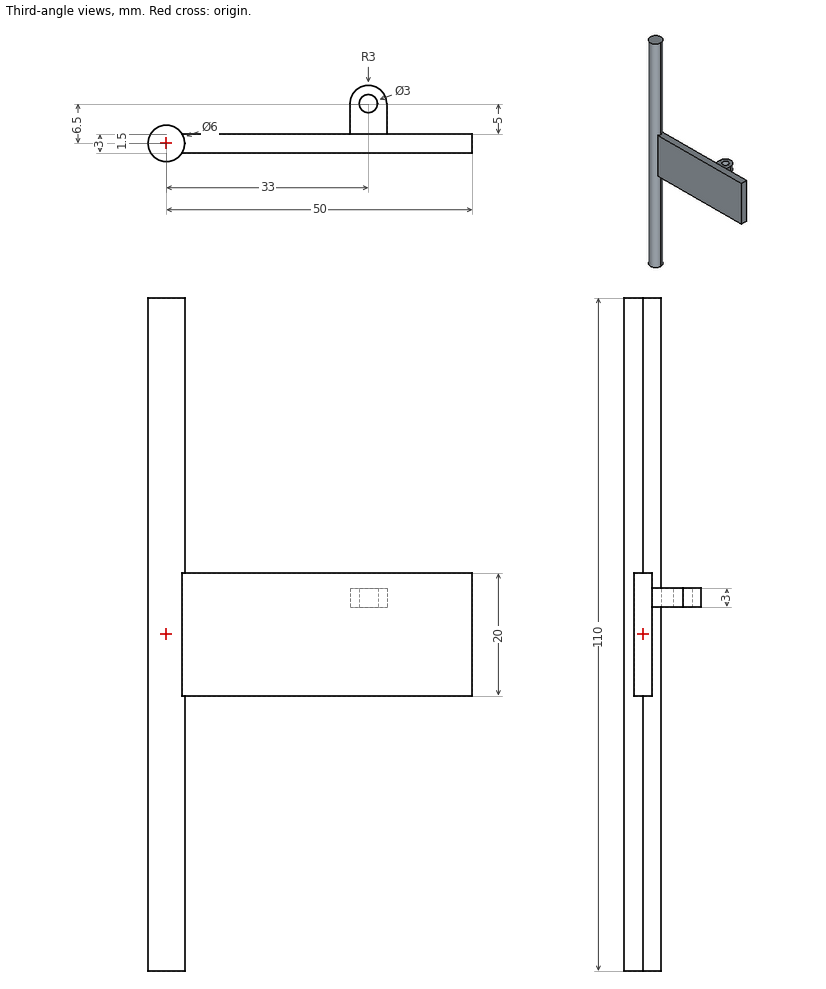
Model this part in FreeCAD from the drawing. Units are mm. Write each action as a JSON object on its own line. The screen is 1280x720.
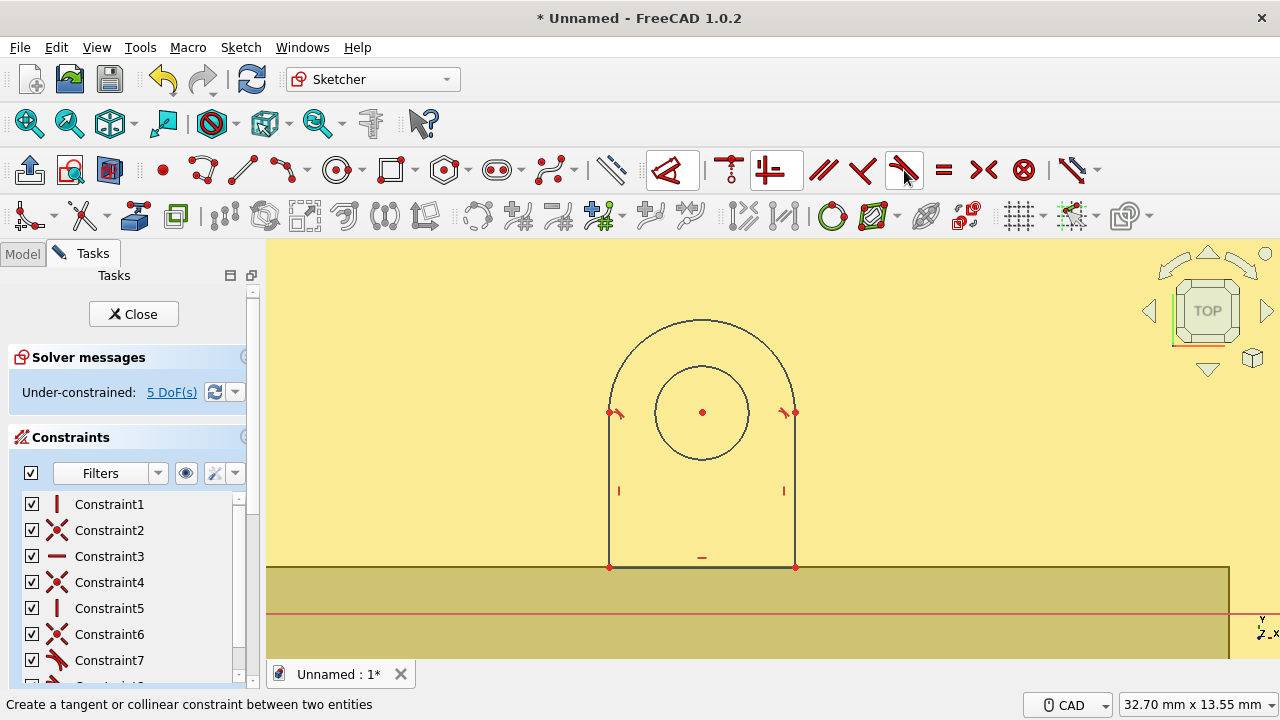
{"action": "left_click", "coordinate": [757, 338]}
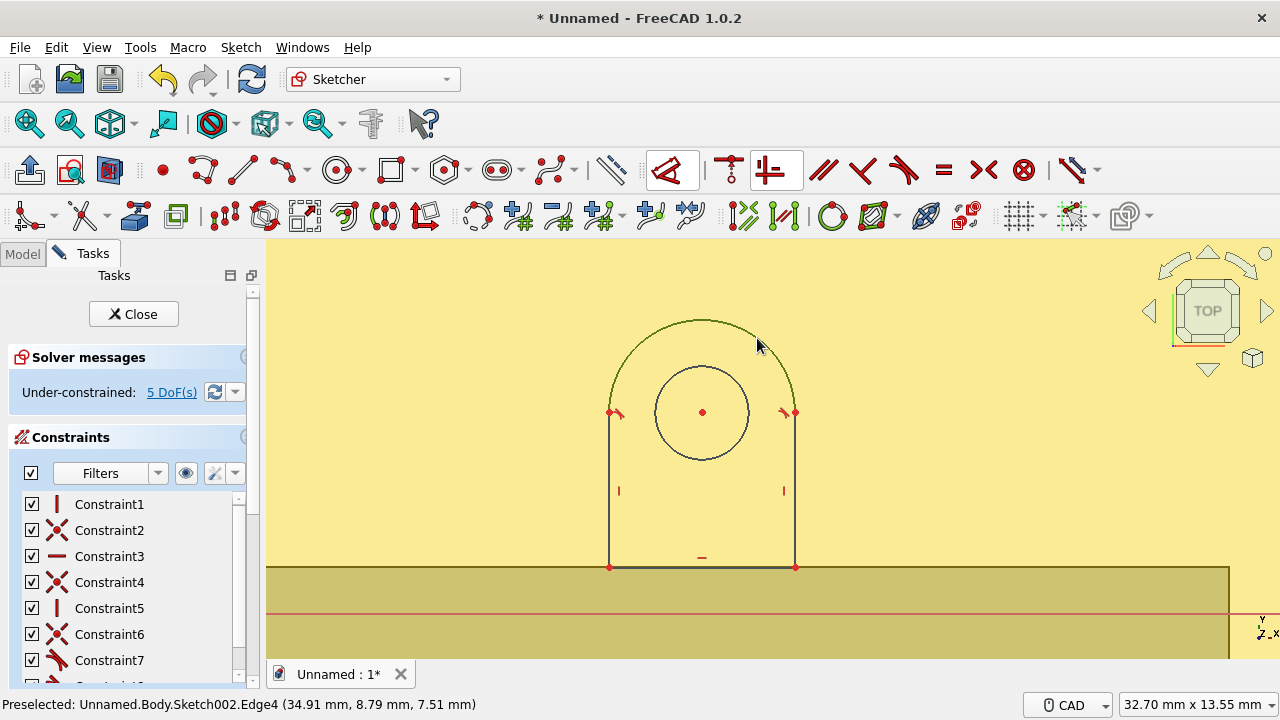
{"action": "left_click", "coordinate": [694, 170]}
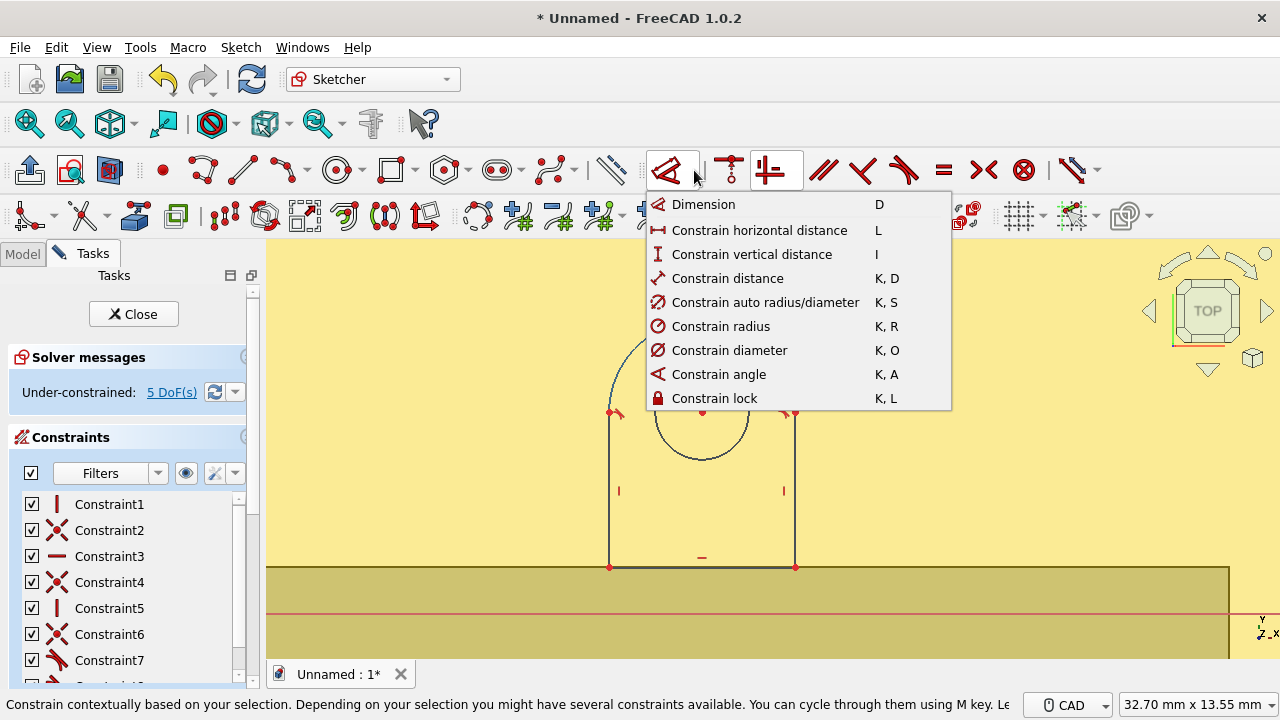
{"action": "left_click", "coordinate": [799, 326]}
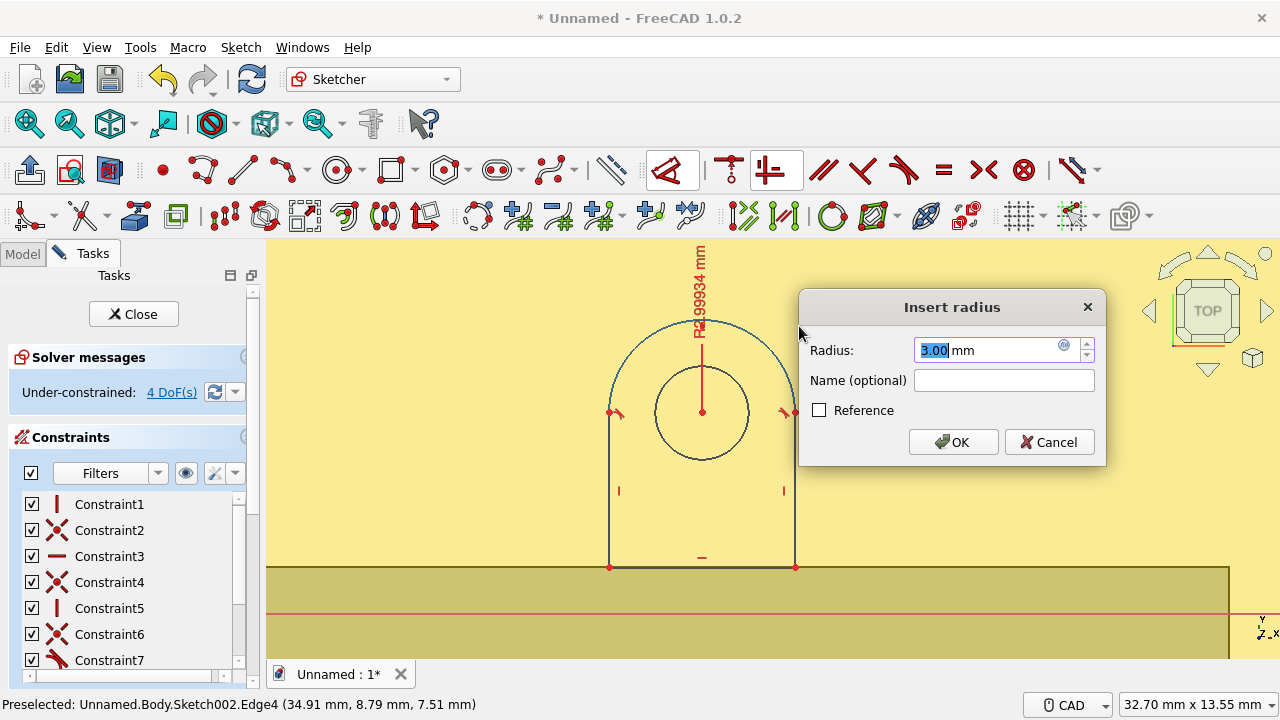
{"action": "type", "text": "3"}
{"action": "key", "text": "Return"}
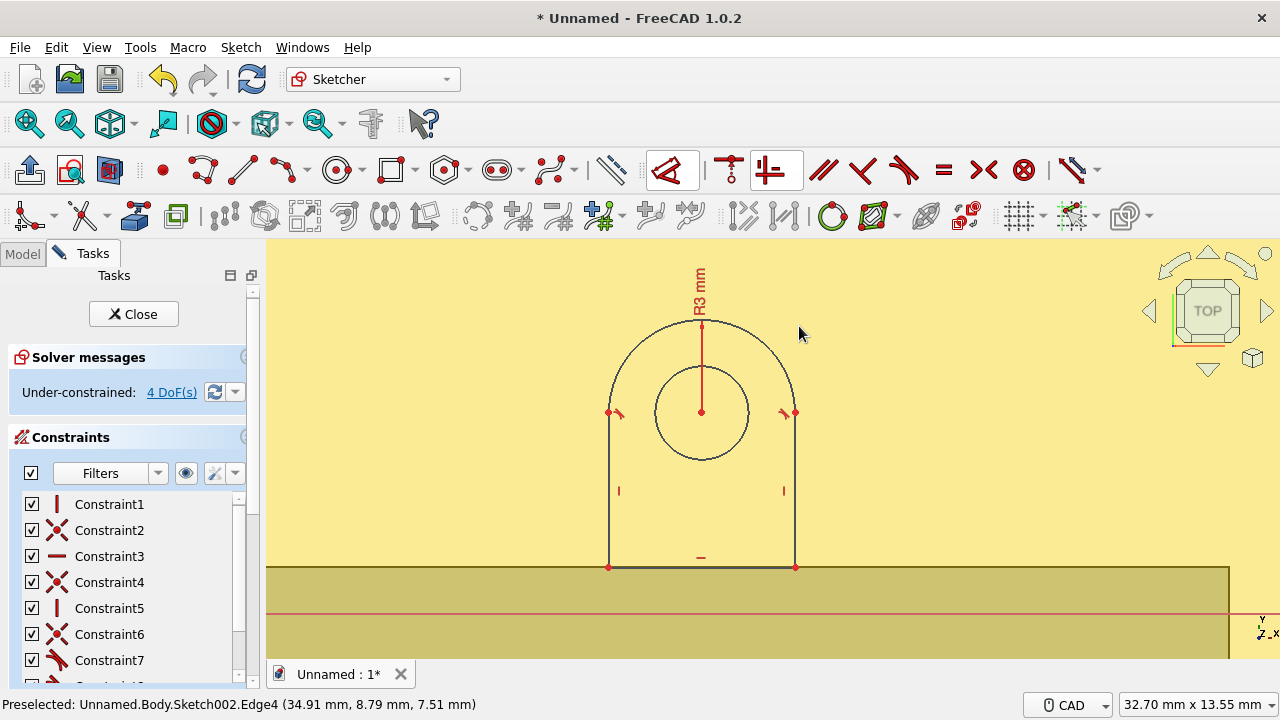
{"action": "left_click", "coordinate": [735, 380]}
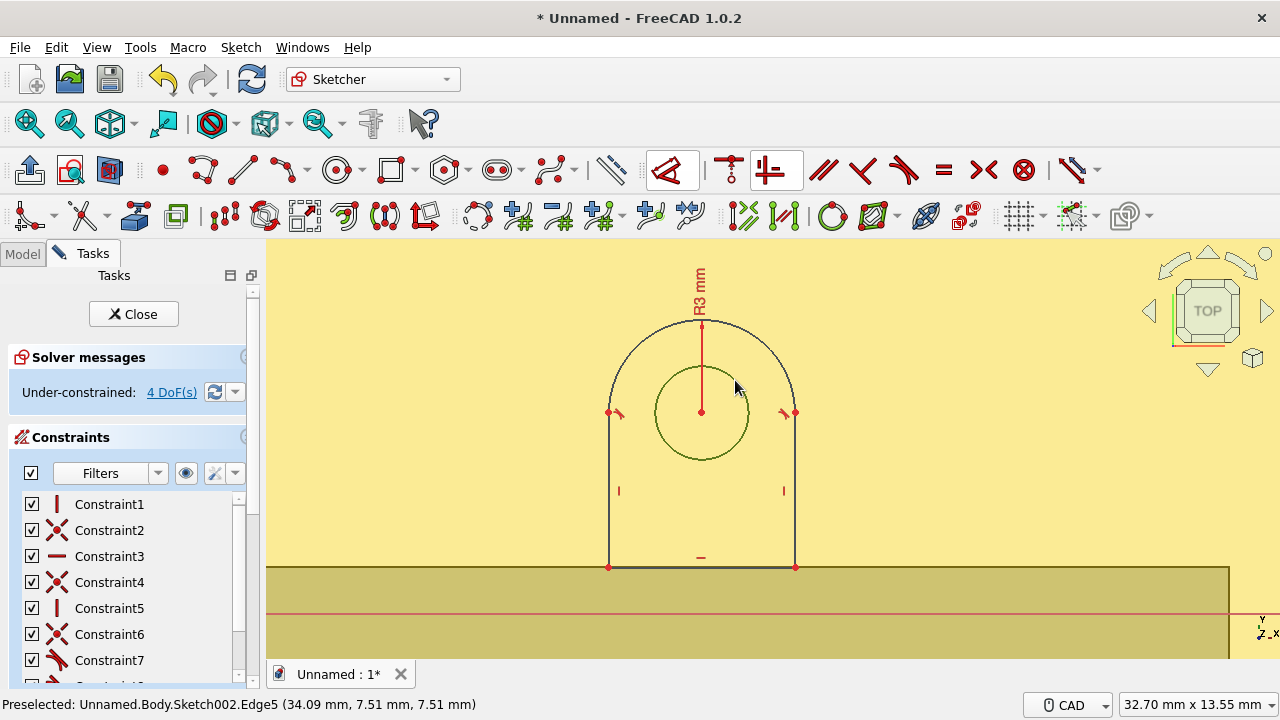
{"action": "left_click", "coordinate": [694, 170]}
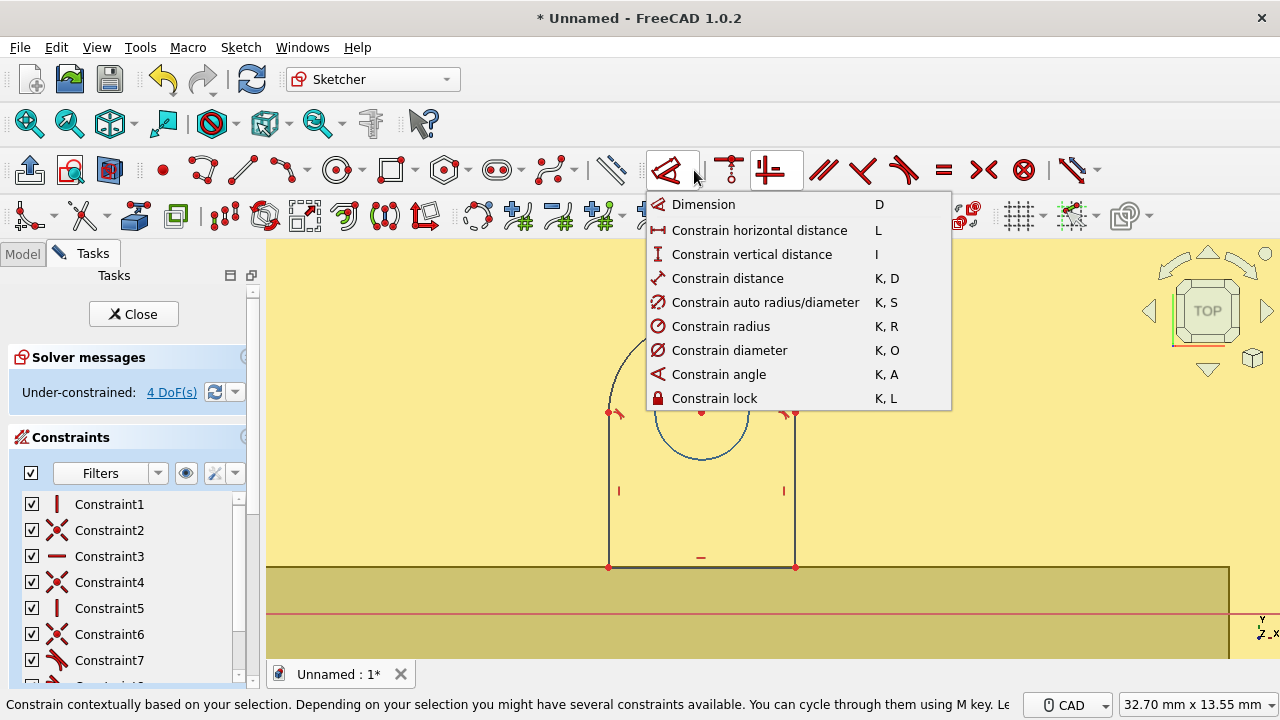
{"action": "left_click", "coordinate": [799, 350]}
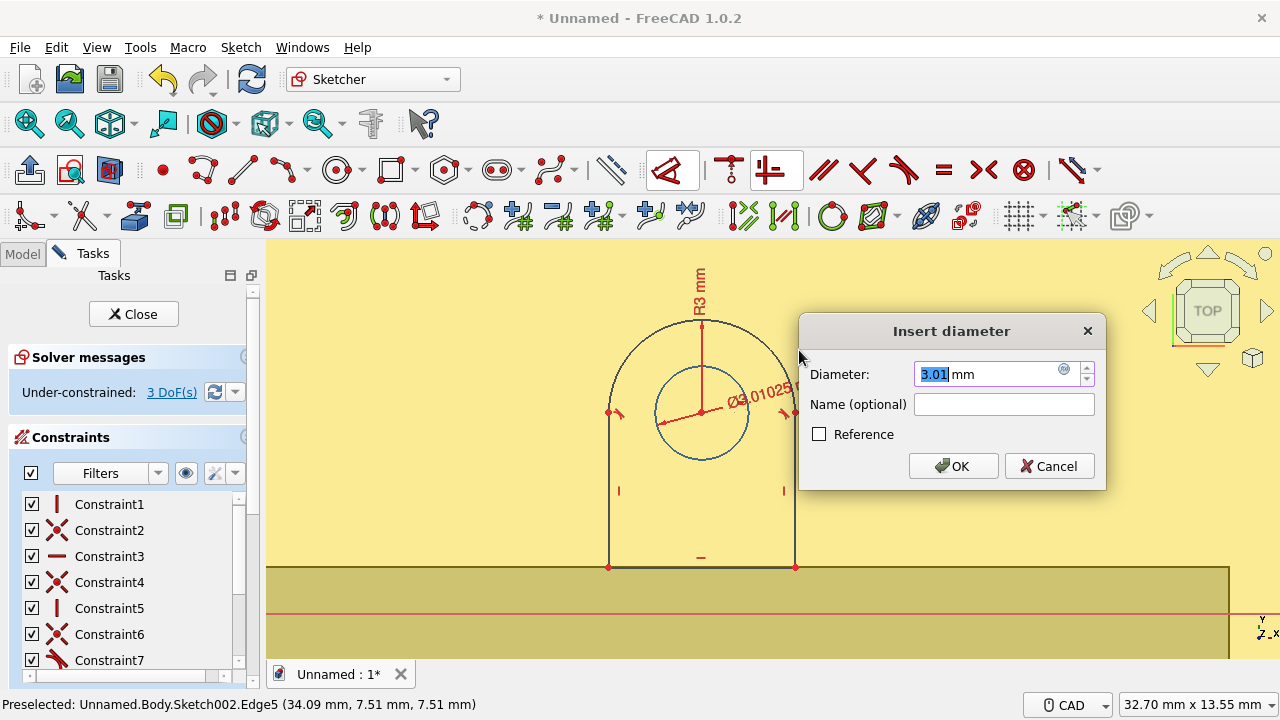
{"action": "type", "text": "3"}
{"action": "key", "text": "Return"}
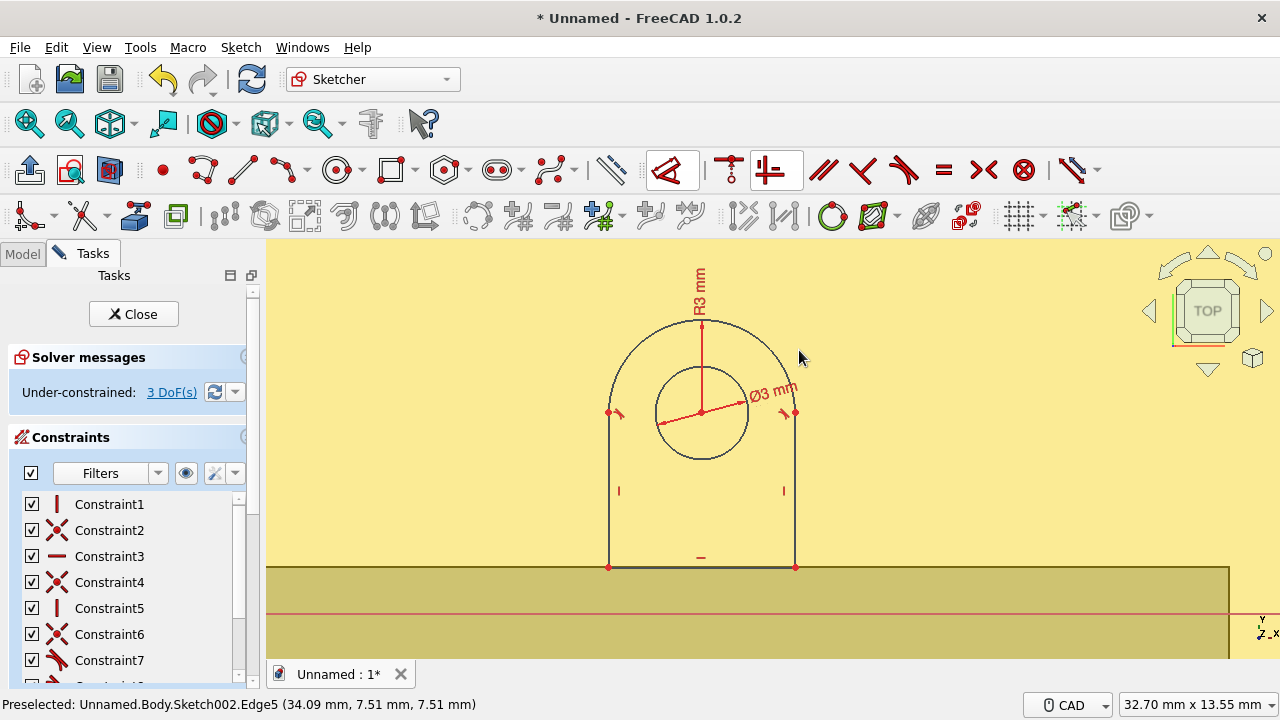
{"action": "left_click", "coordinate": [609, 460]}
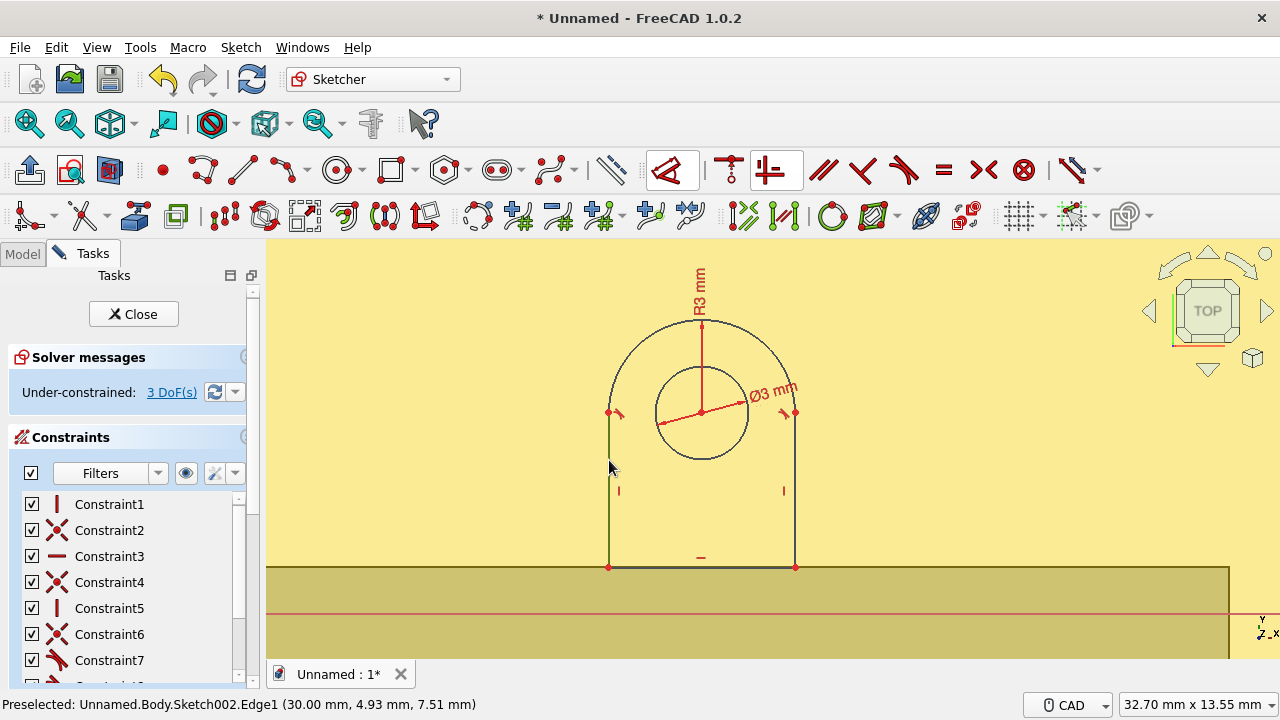
{"action": "left_click", "coordinate": [694, 170]}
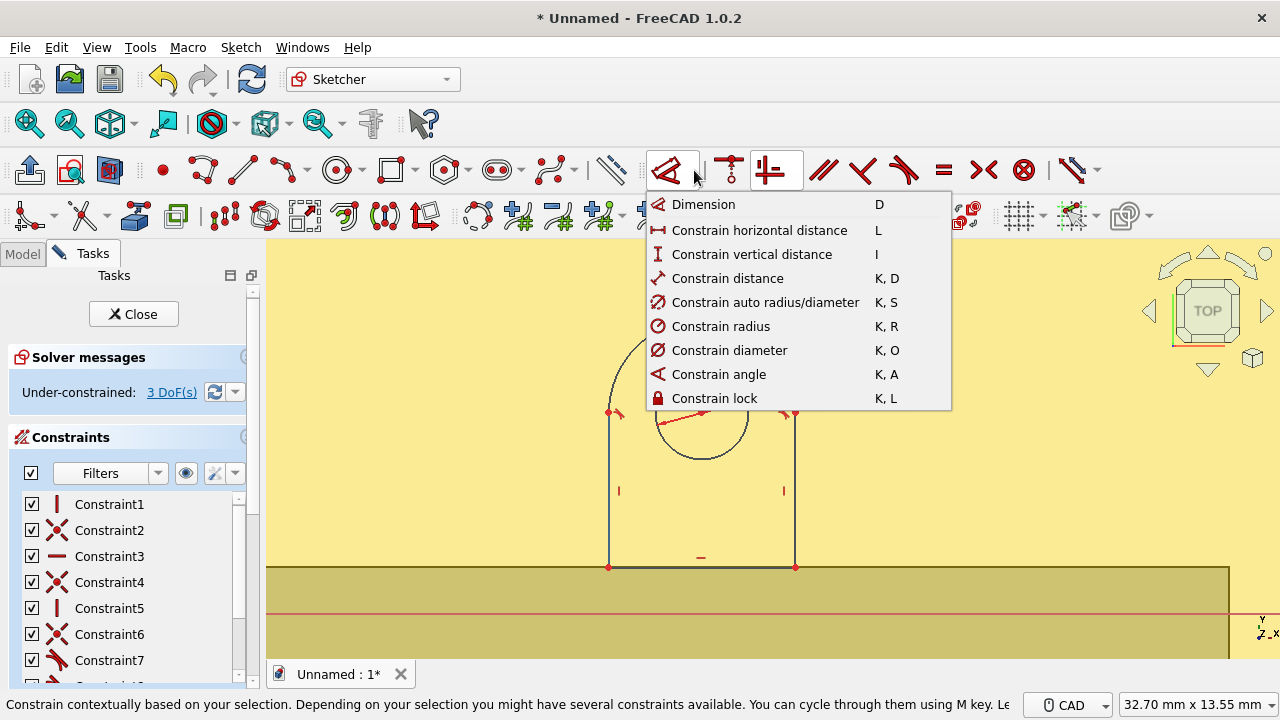
{"action": "left_click", "coordinate": [799, 254]}